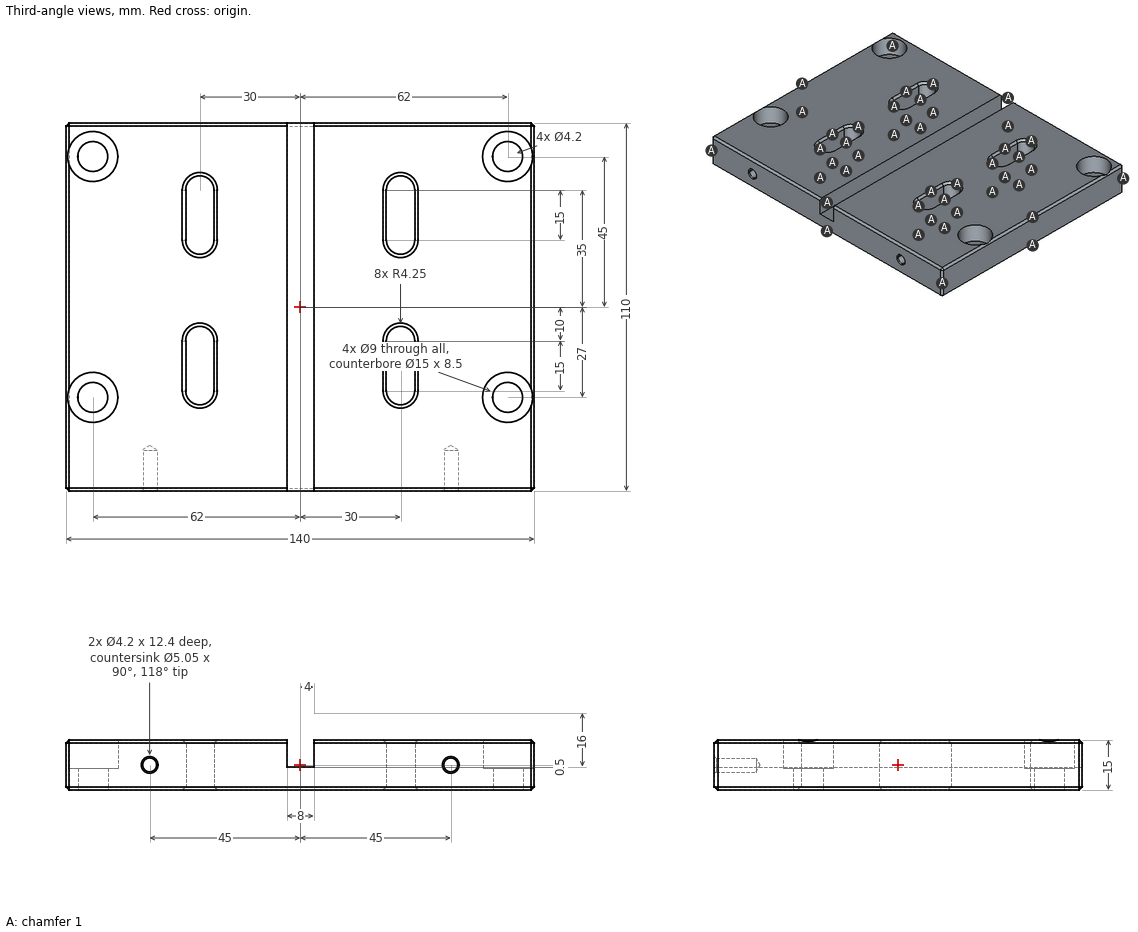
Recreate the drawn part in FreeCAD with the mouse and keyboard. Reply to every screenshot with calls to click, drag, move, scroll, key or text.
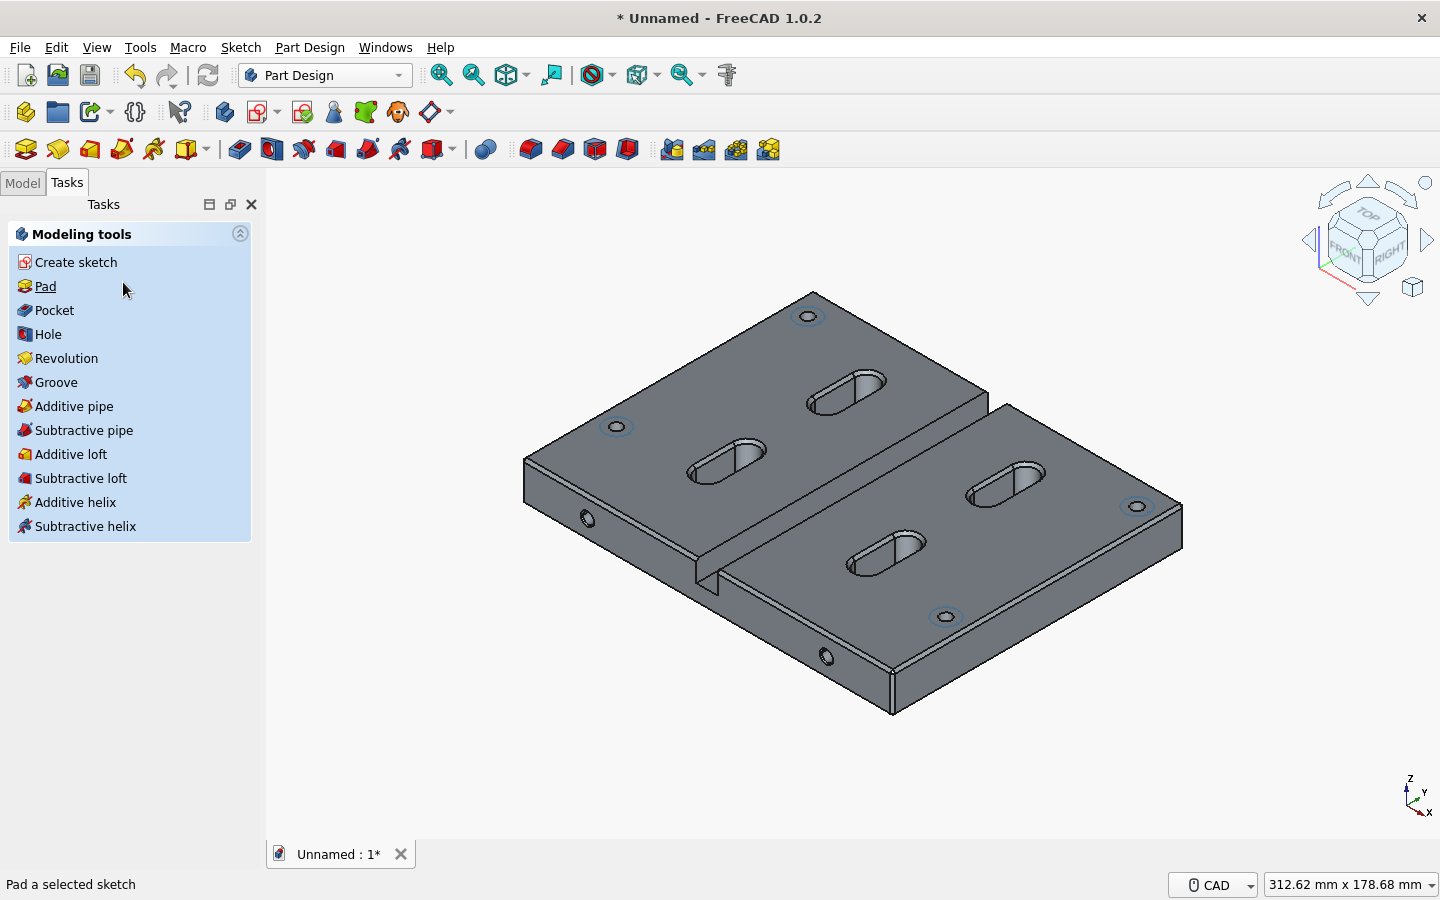
click(272, 150)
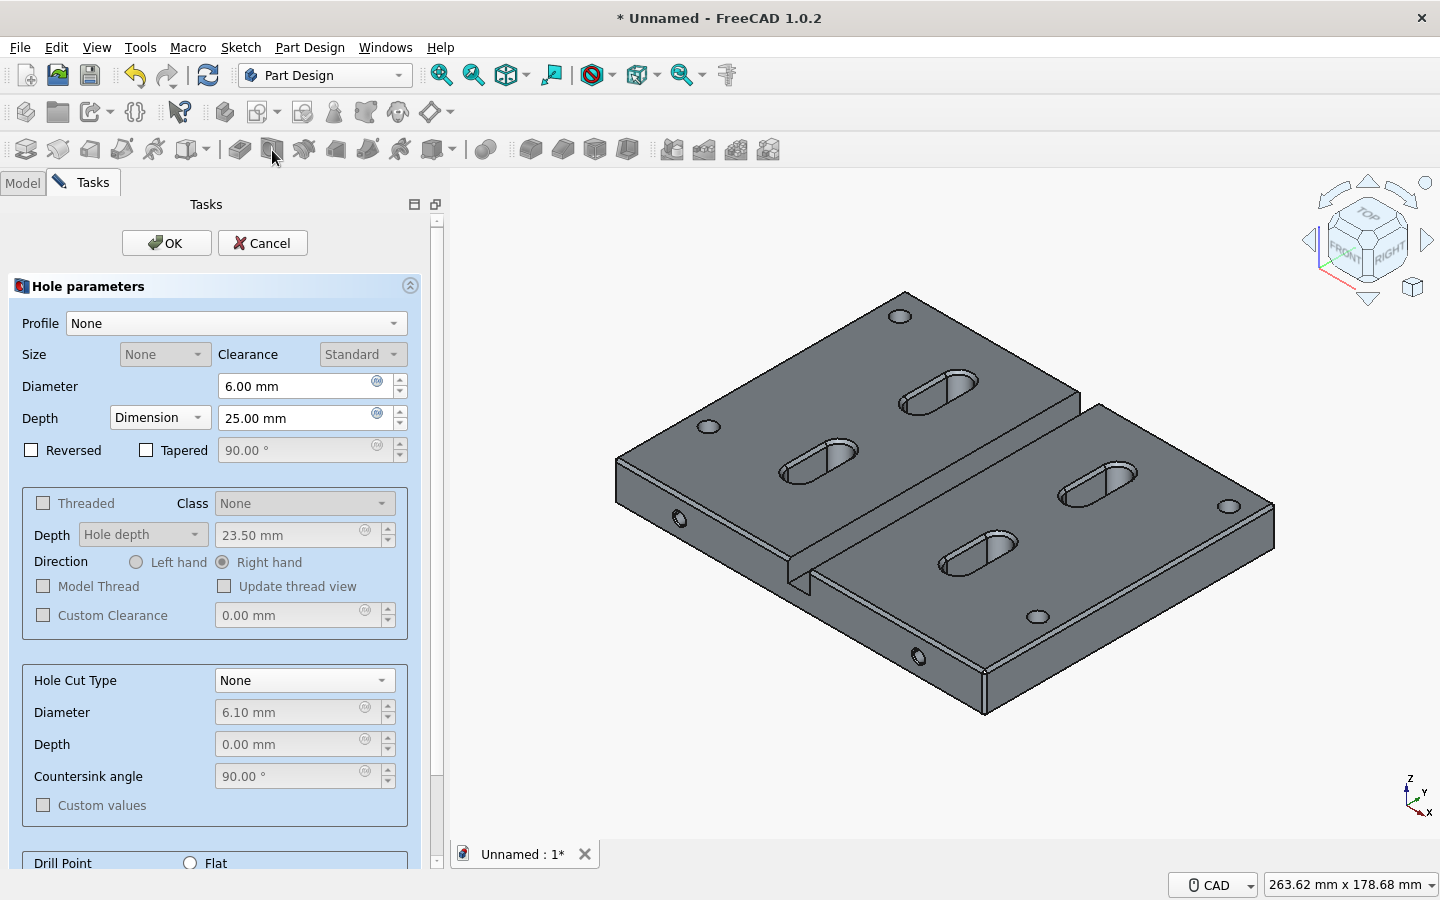
triple_click(305, 386)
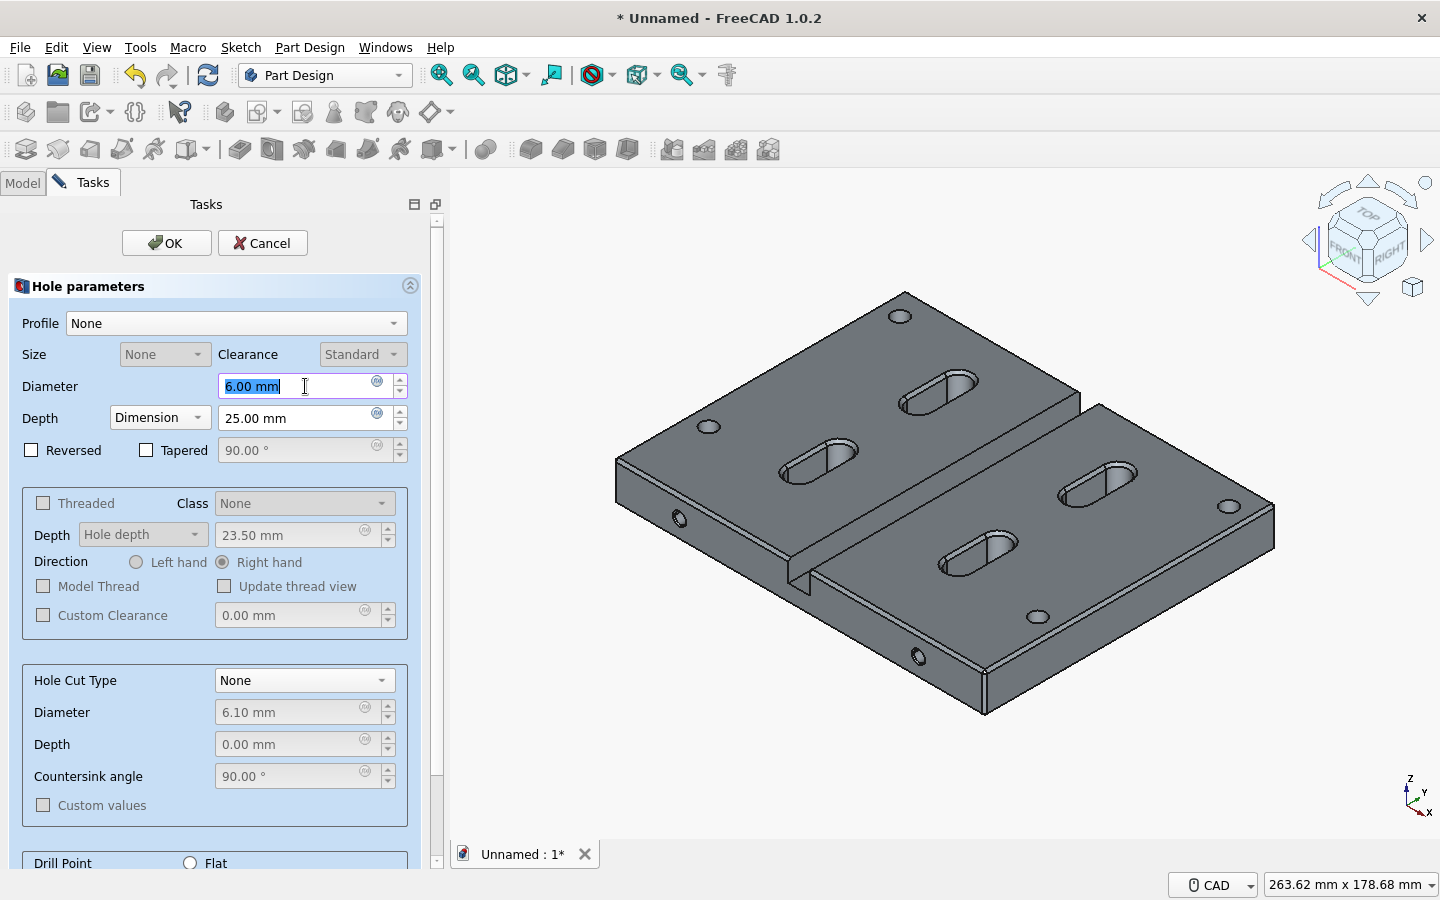
text(9)
key(Tab)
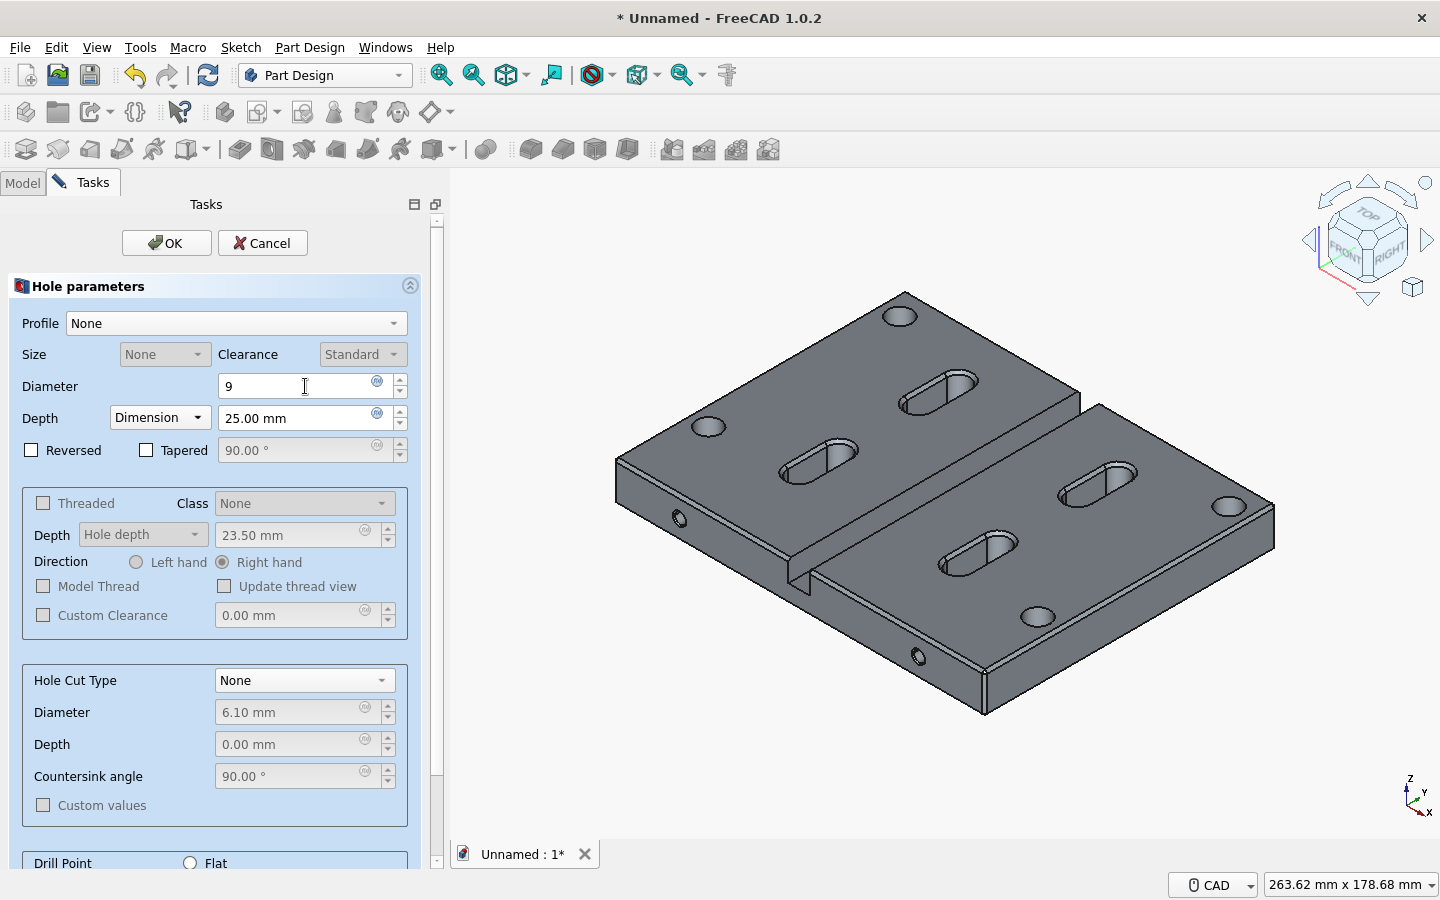
click(161, 418)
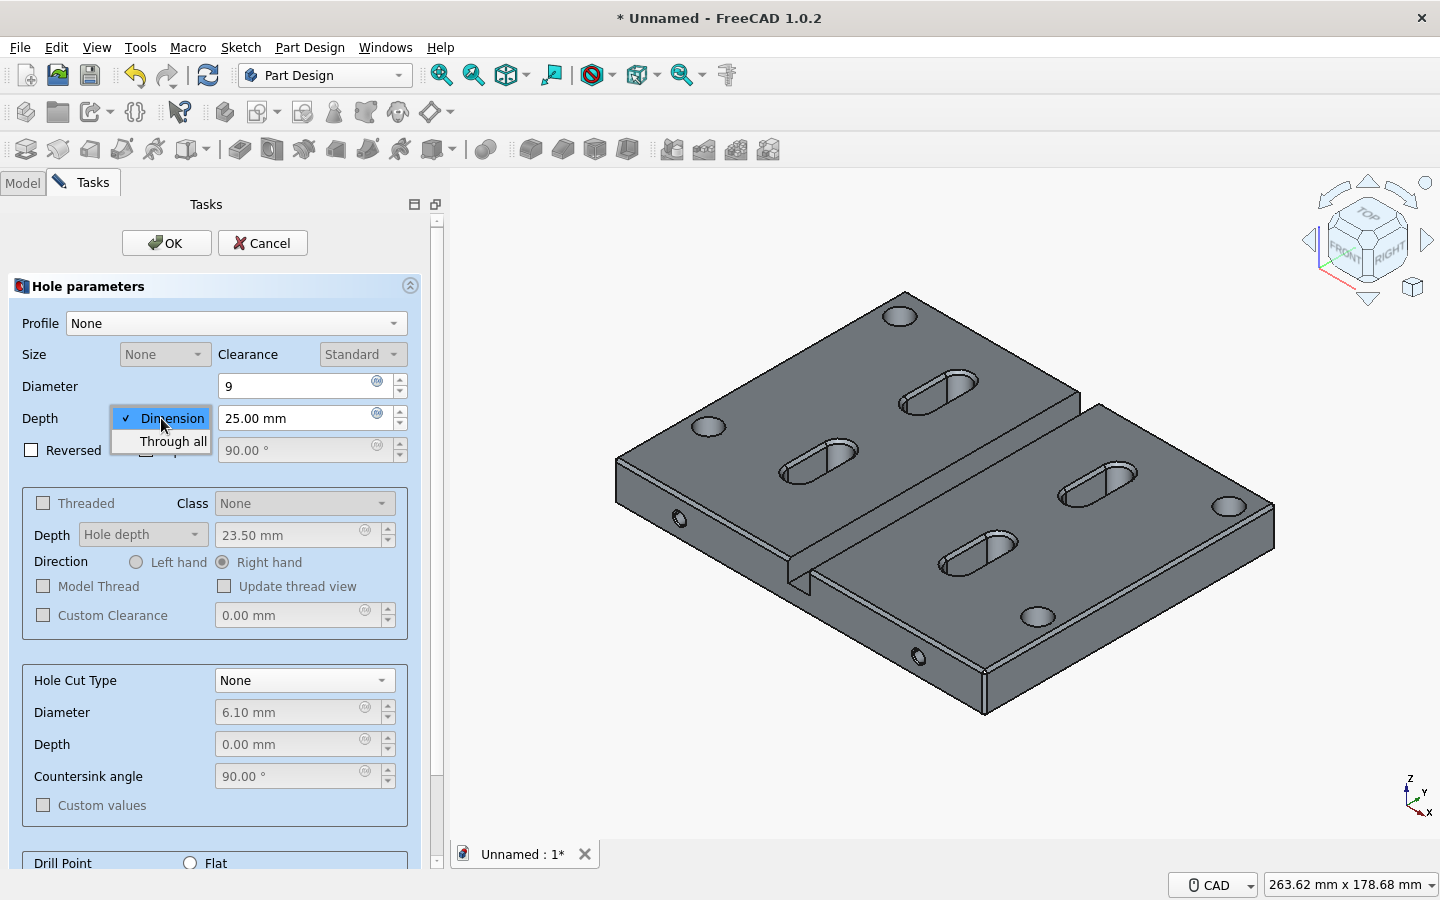
click(160, 442)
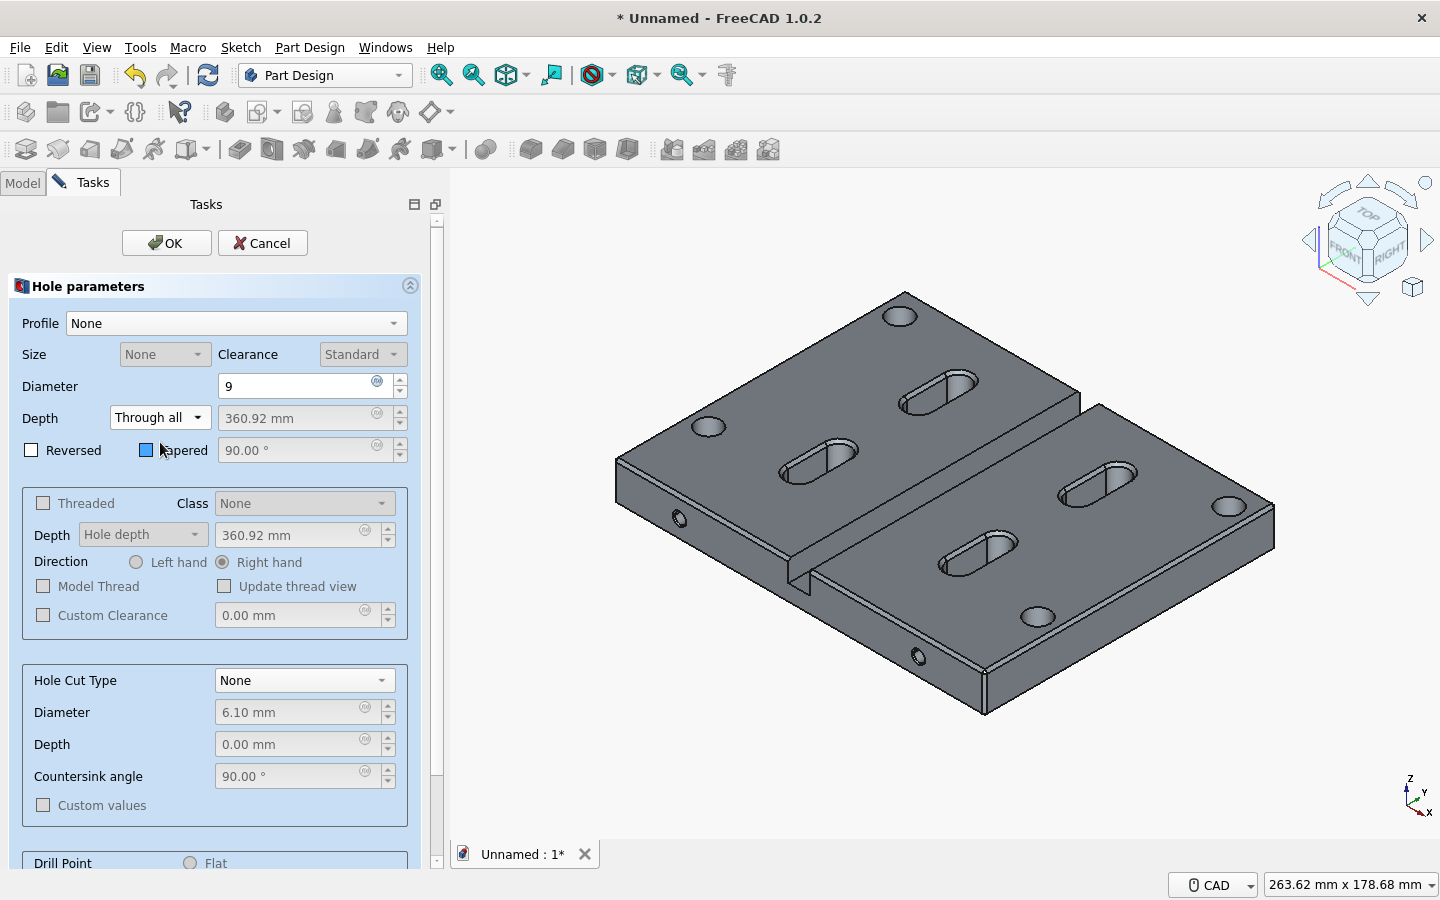
click(306, 680)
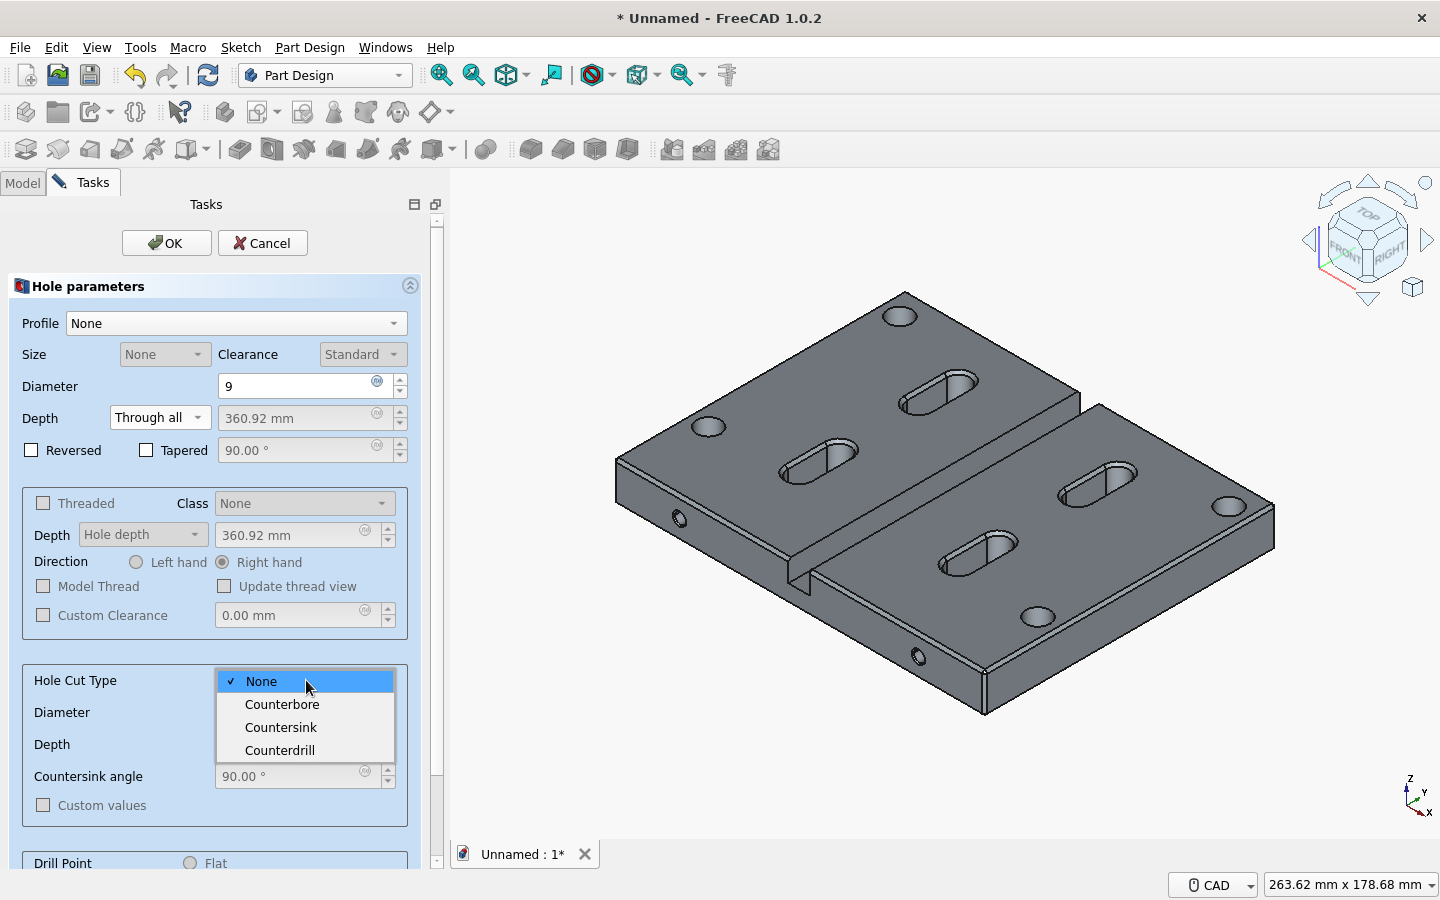
click(304, 704)